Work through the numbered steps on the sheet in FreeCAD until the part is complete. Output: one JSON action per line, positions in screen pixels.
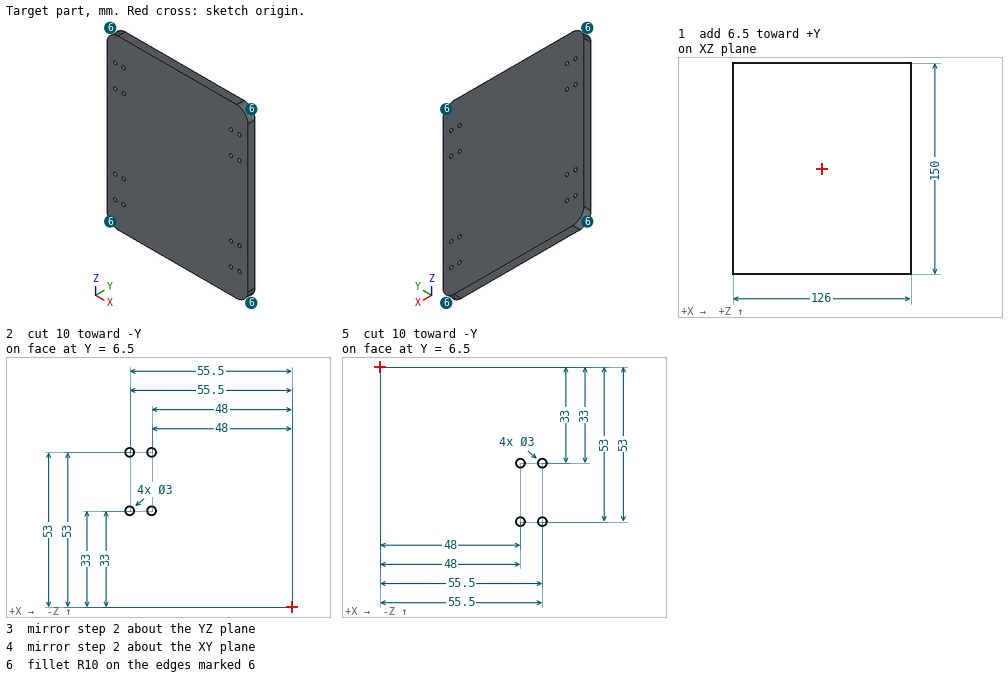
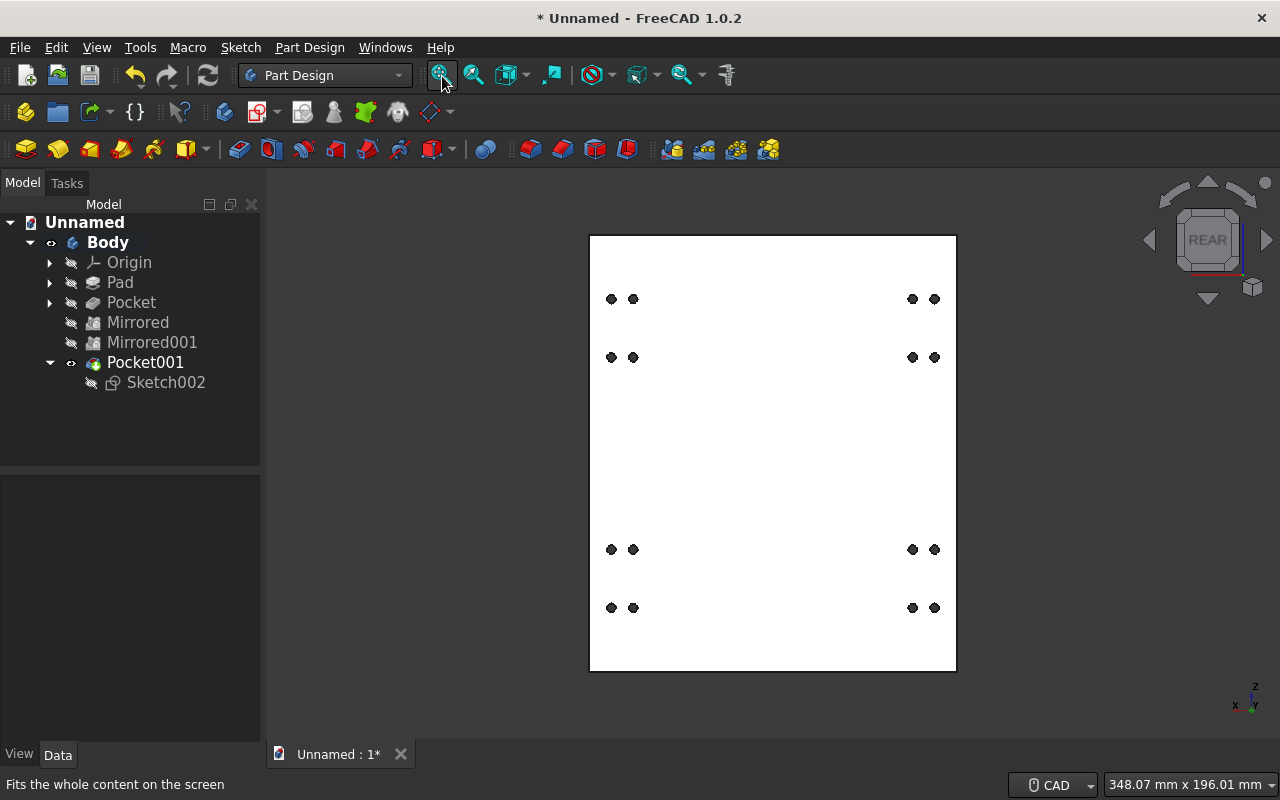
{"action": "key", "text": "0"}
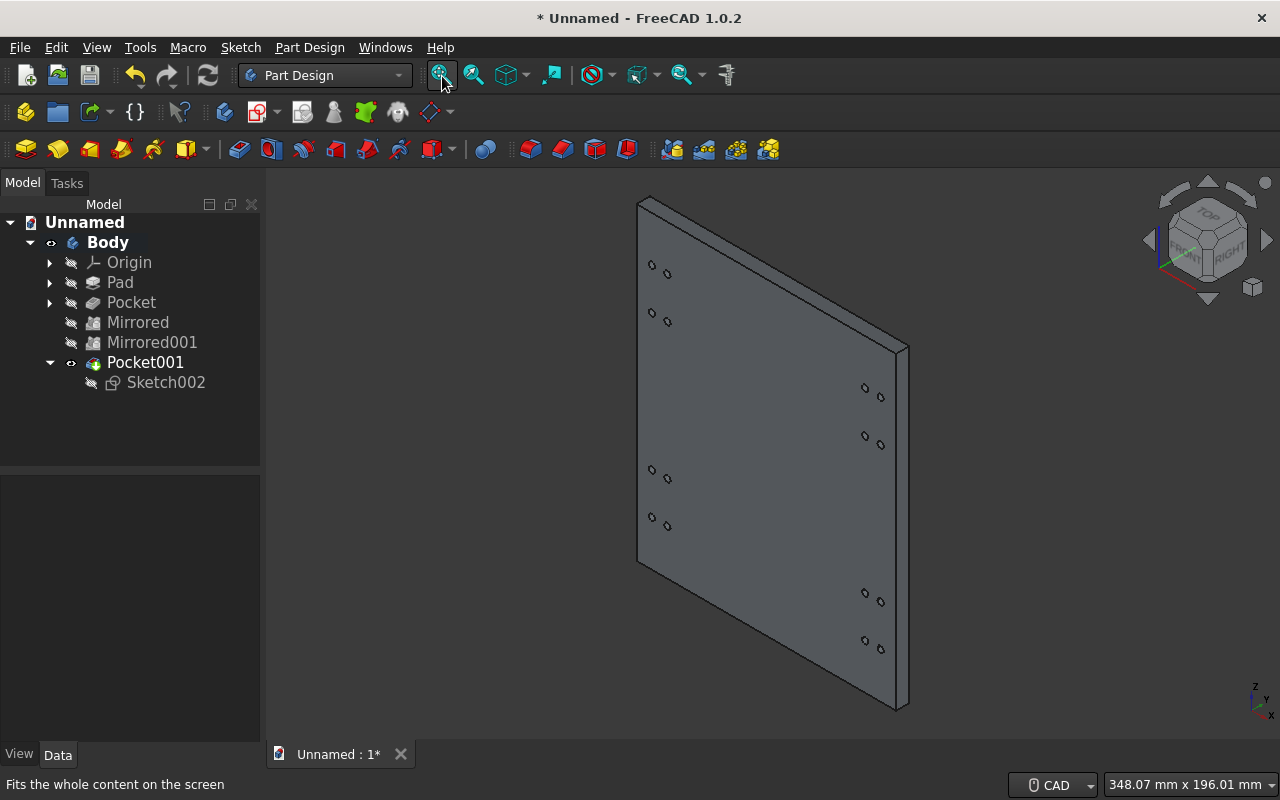
{"action": "left_click", "coordinate": [903, 349]}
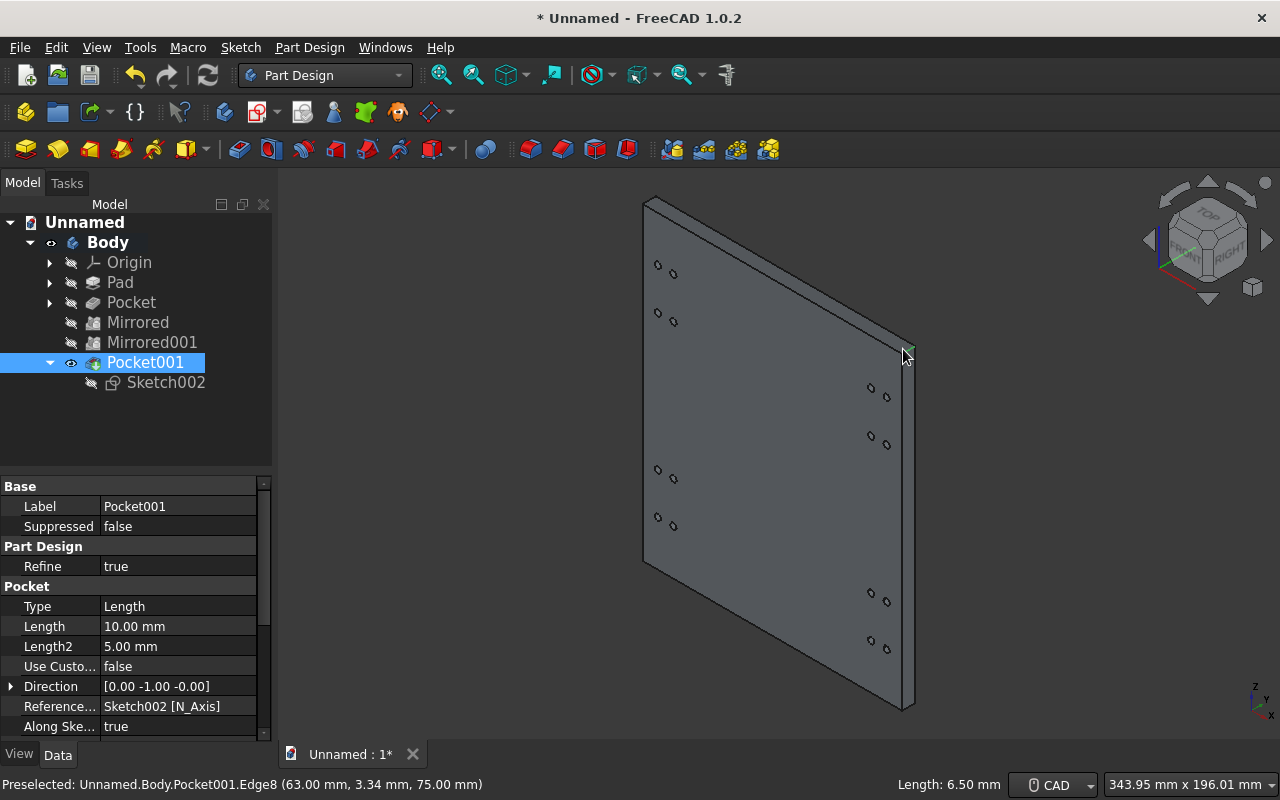
{"action": "scroll", "coordinate": [649, 199], "scroll_direction": "up", "scroll_amount": 4}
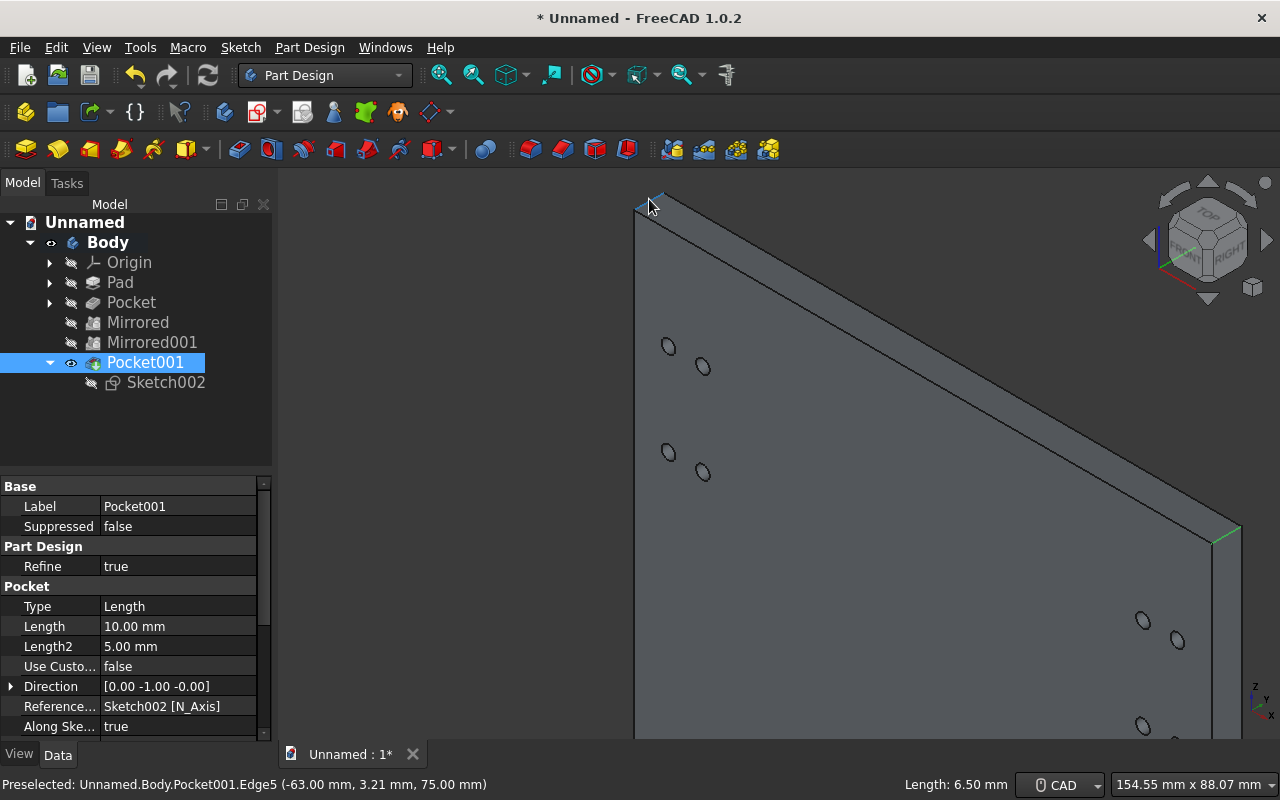
{"action": "left_click", "coordinate": [442, 76]}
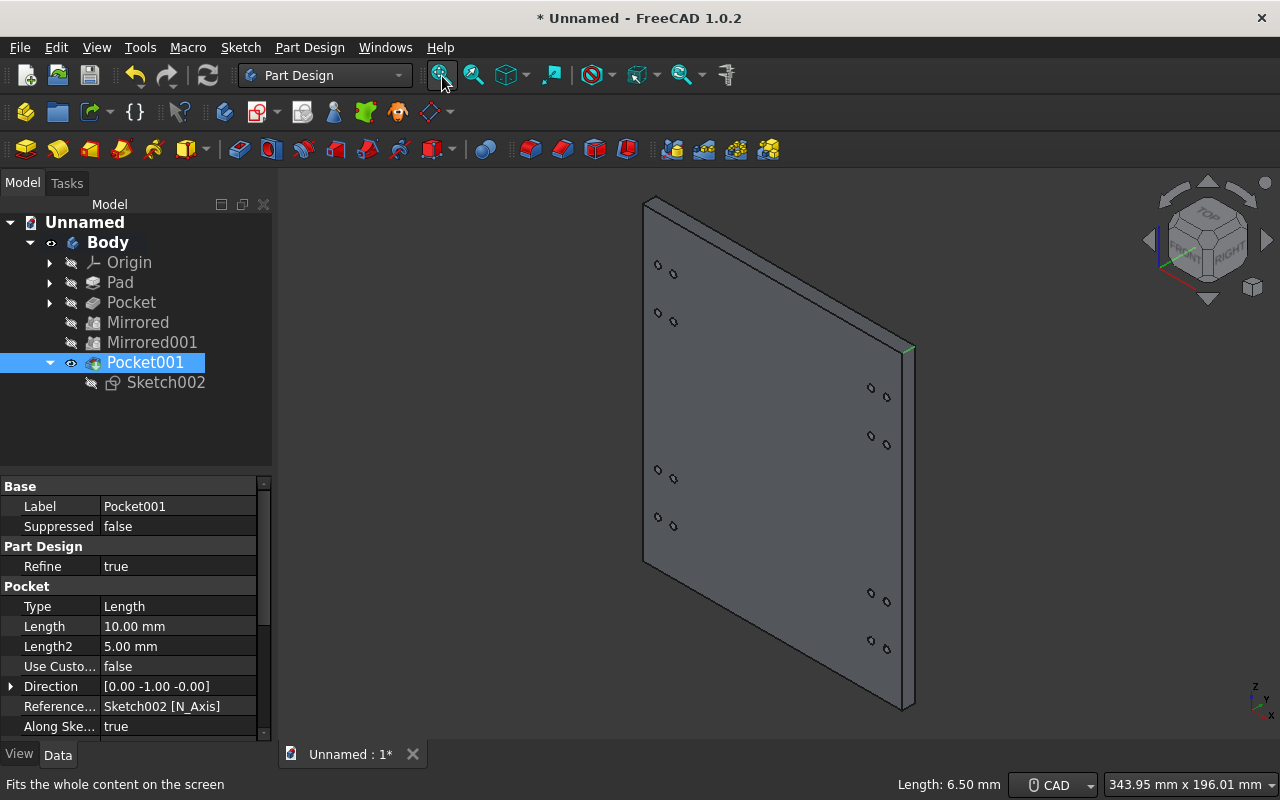
{"action": "key", "text": "2"}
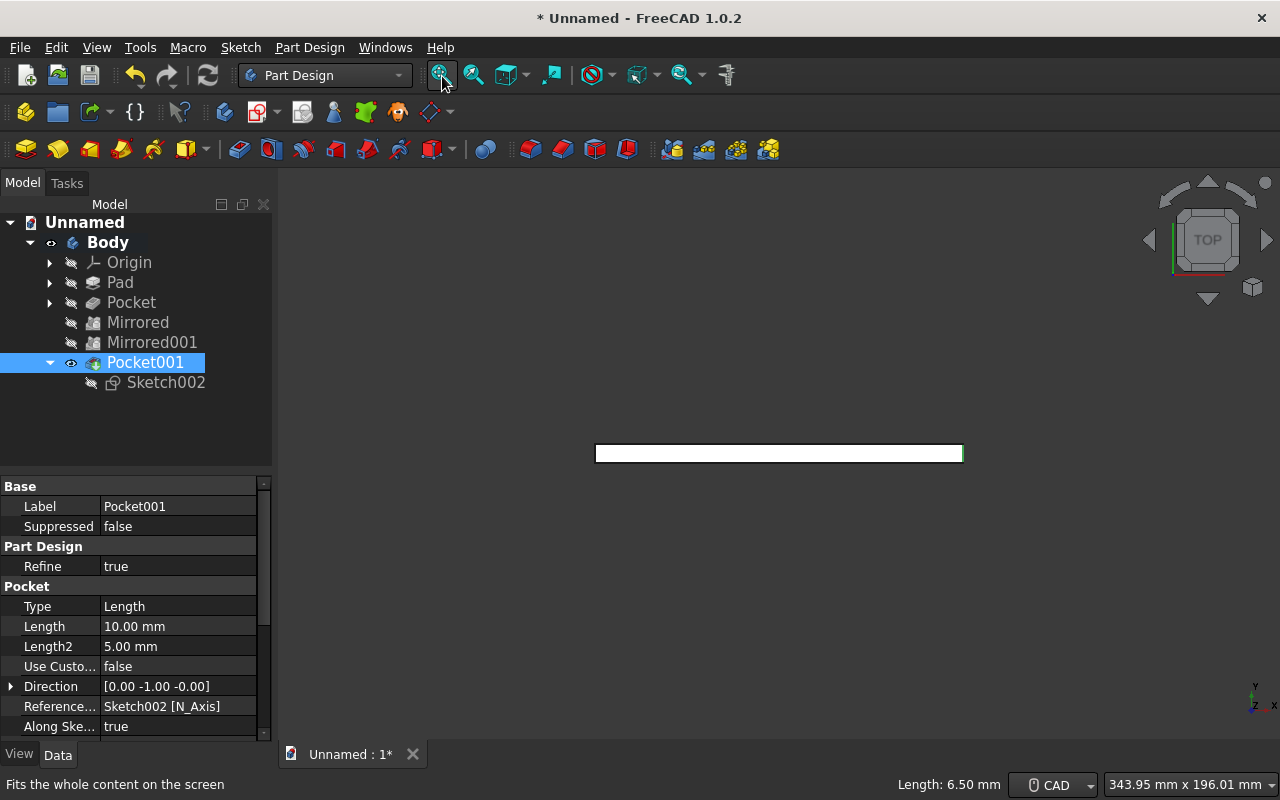
{"action": "left_click", "coordinate": [442, 76]}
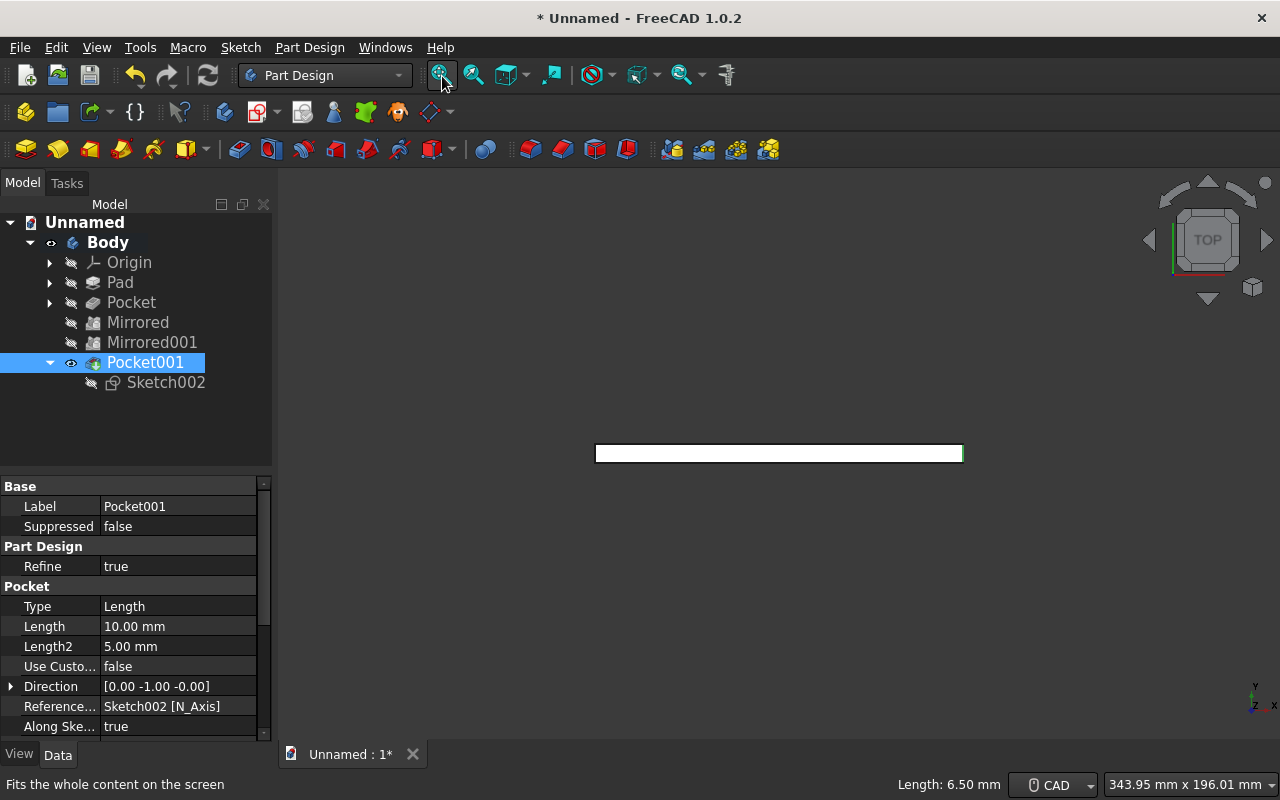
{"action": "left_click", "coordinate": [595, 452], "text": "ctrl"}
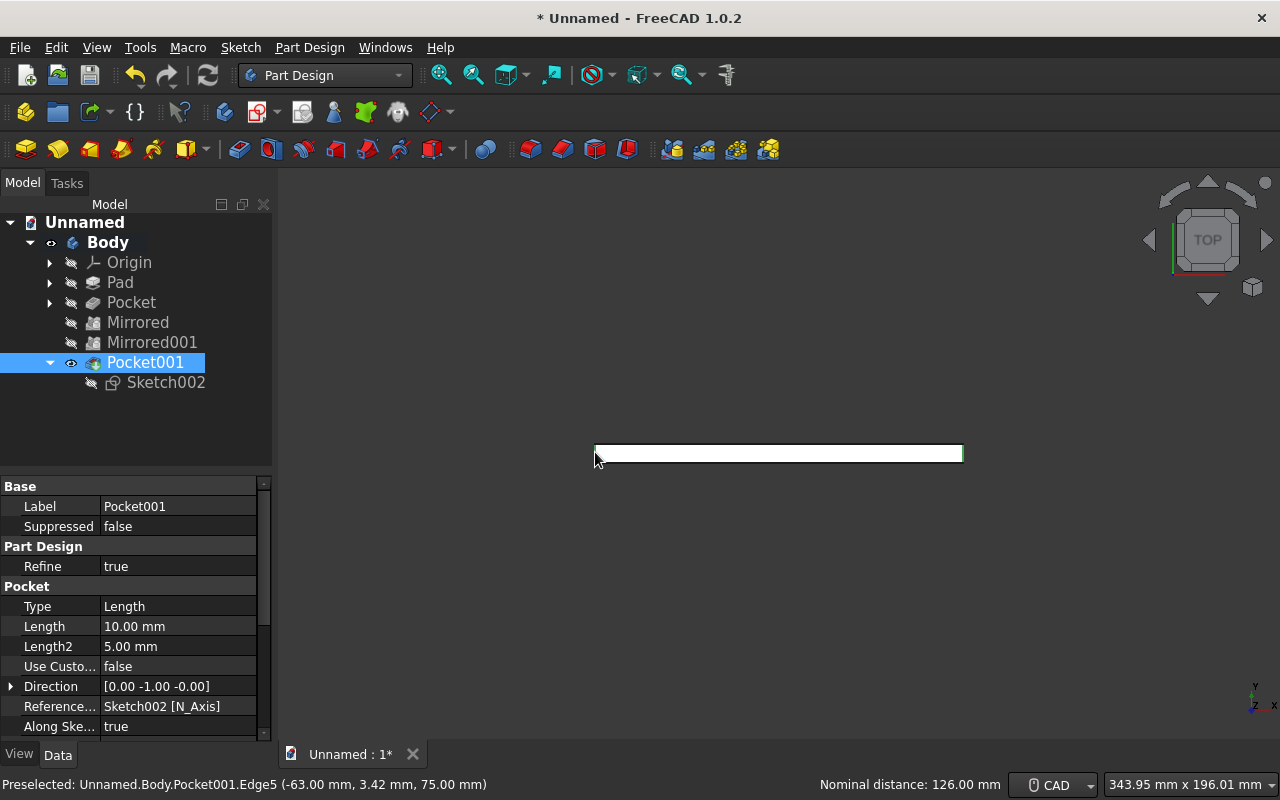
{"action": "scroll", "coordinate": [595, 452], "scroll_direction": "up", "scroll_amount": 4}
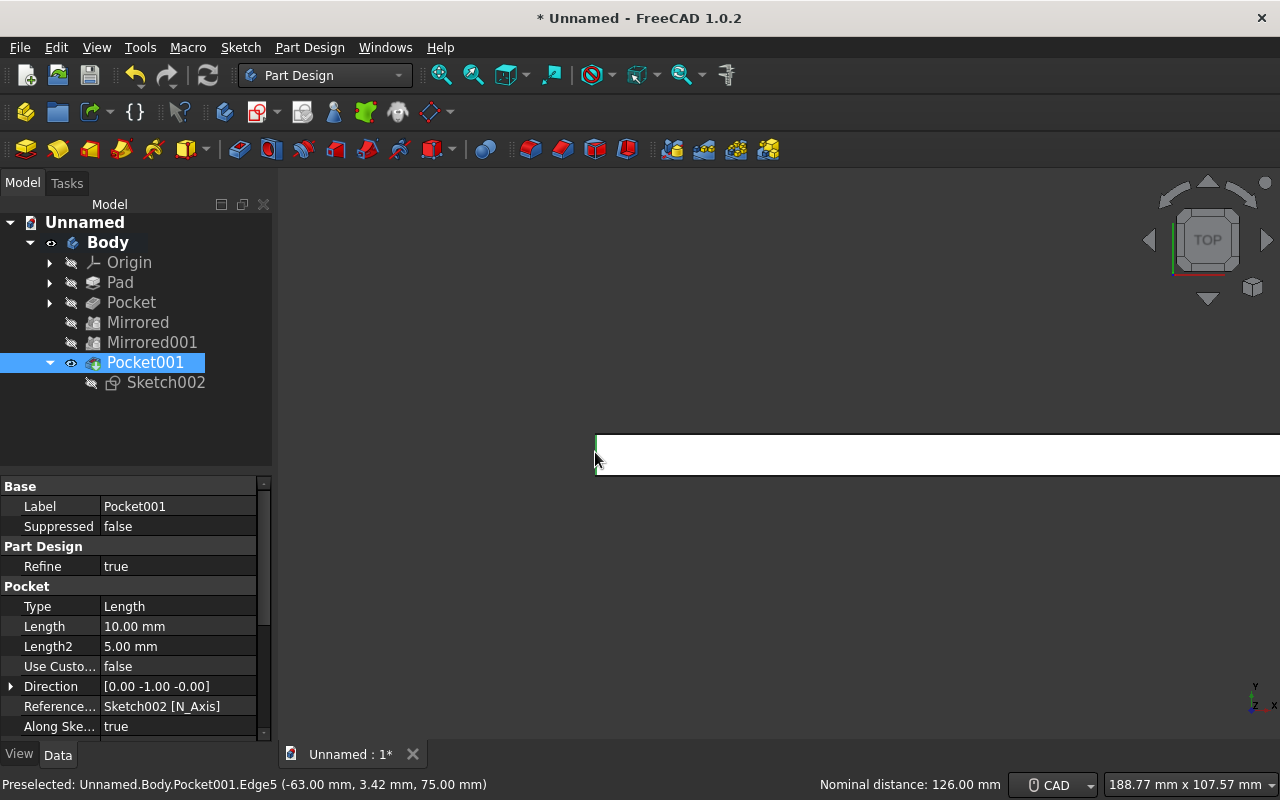
{"action": "left_click", "coordinate": [442, 76]}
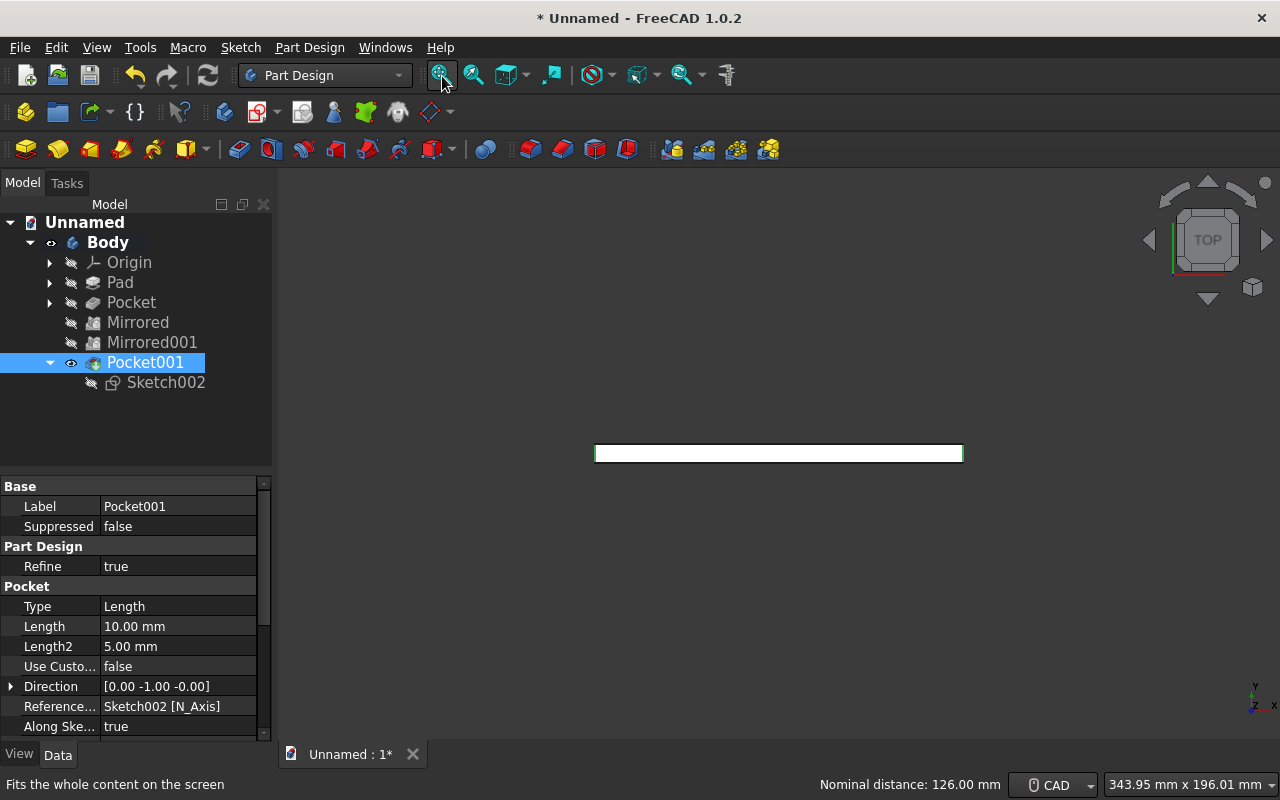
{"action": "key", "text": "1"}